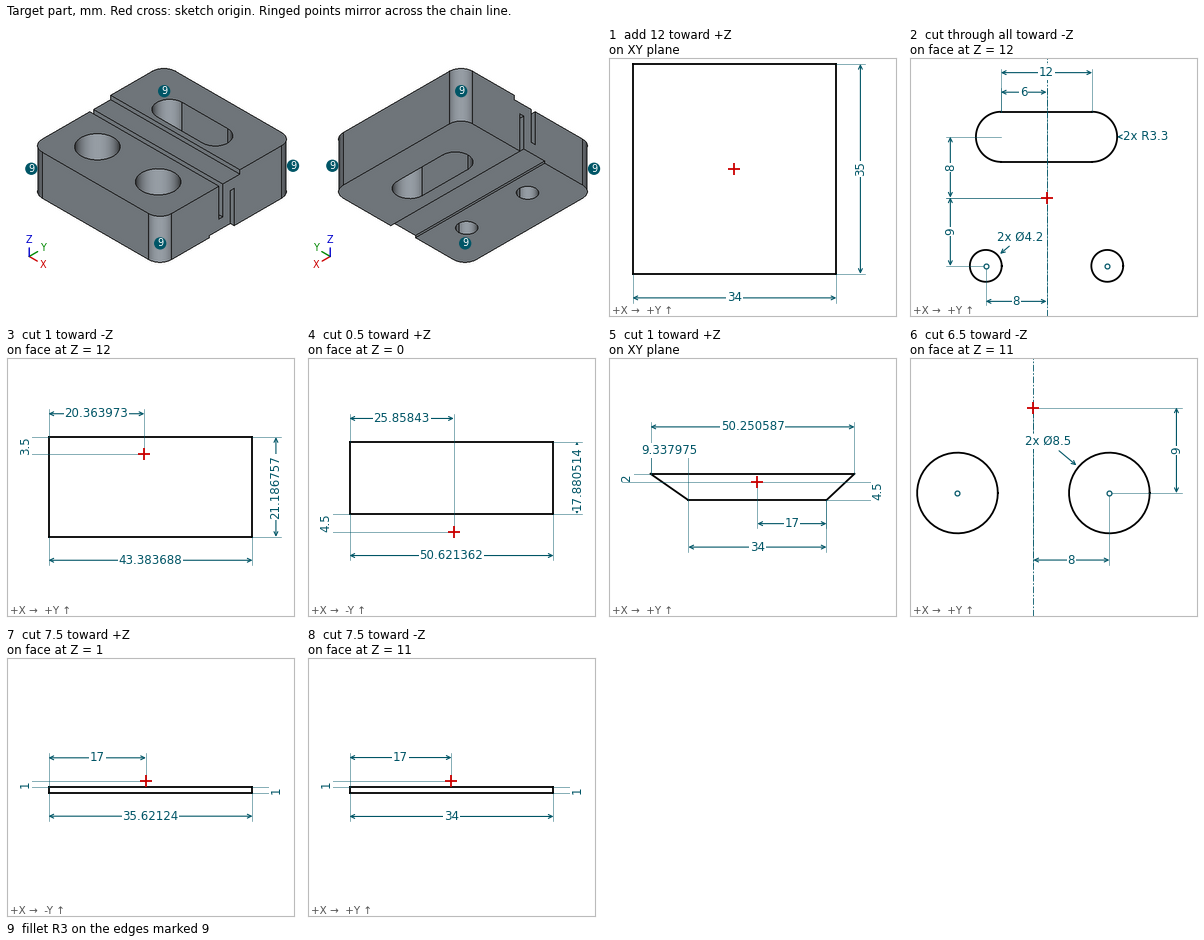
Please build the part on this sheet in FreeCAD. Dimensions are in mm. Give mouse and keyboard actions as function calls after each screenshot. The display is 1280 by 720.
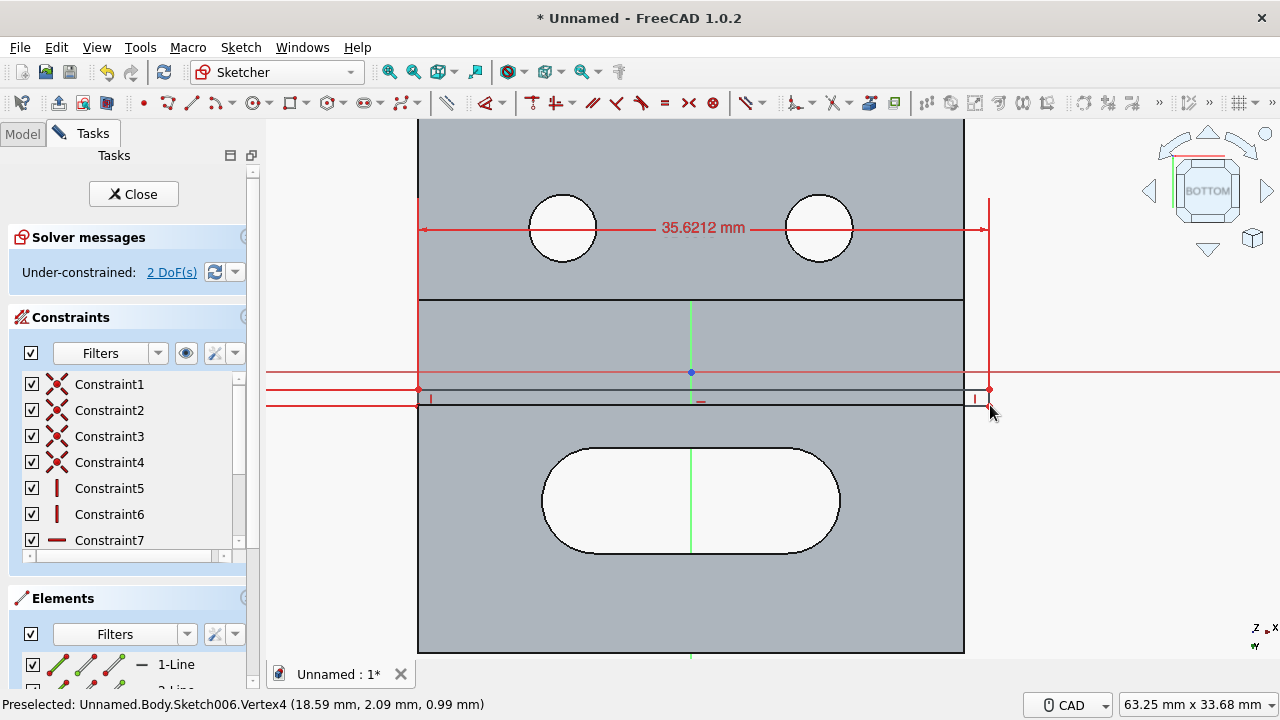
click(486, 104)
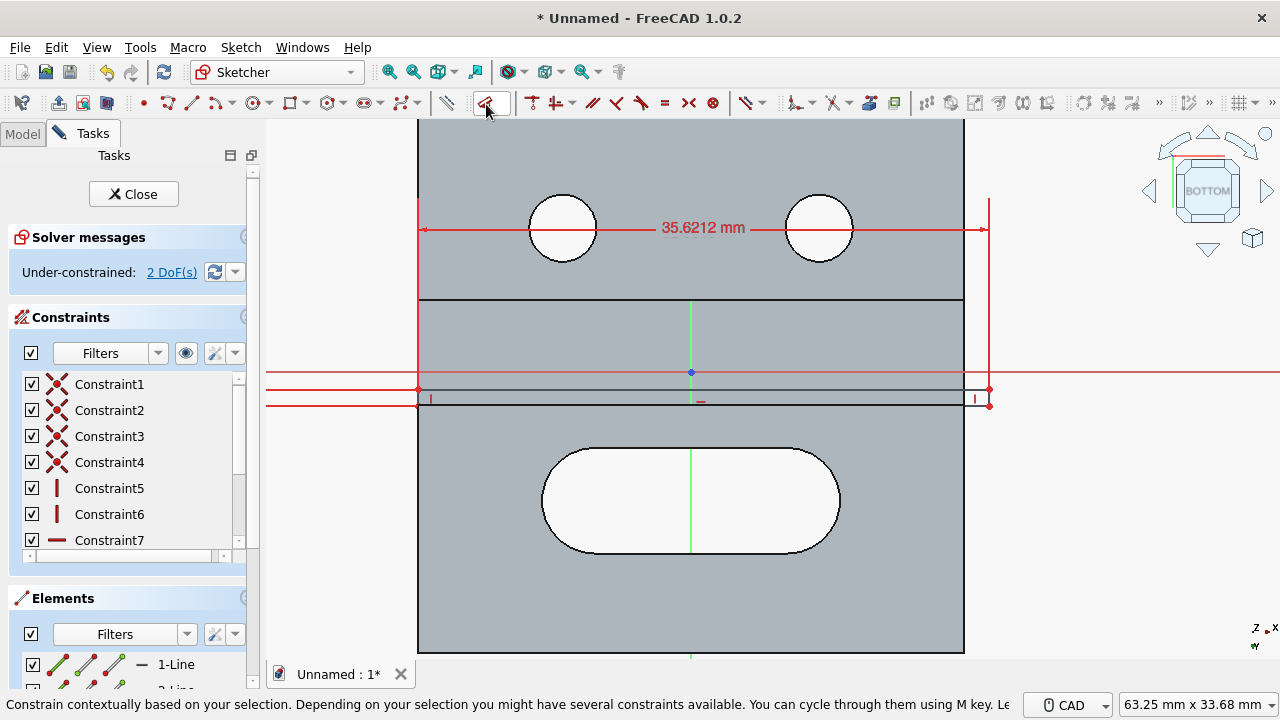
scroll(418, 390, up, 5)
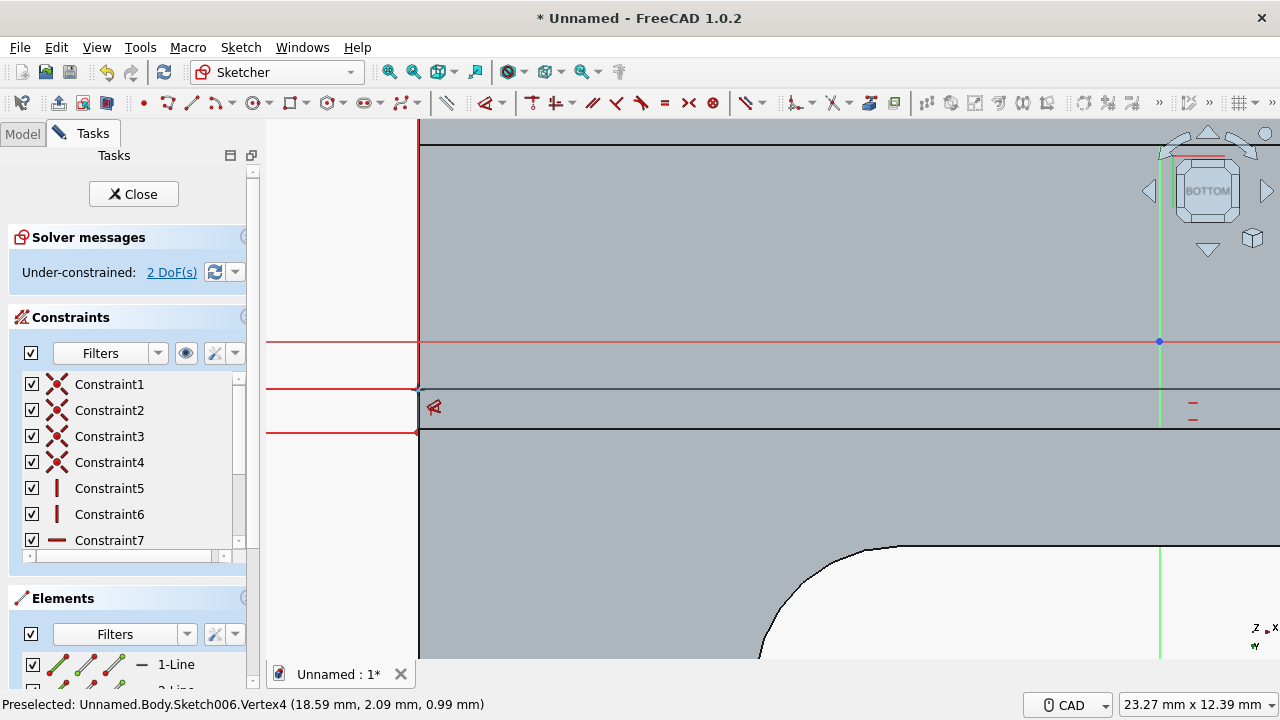
click(418, 389)
click(384, 365)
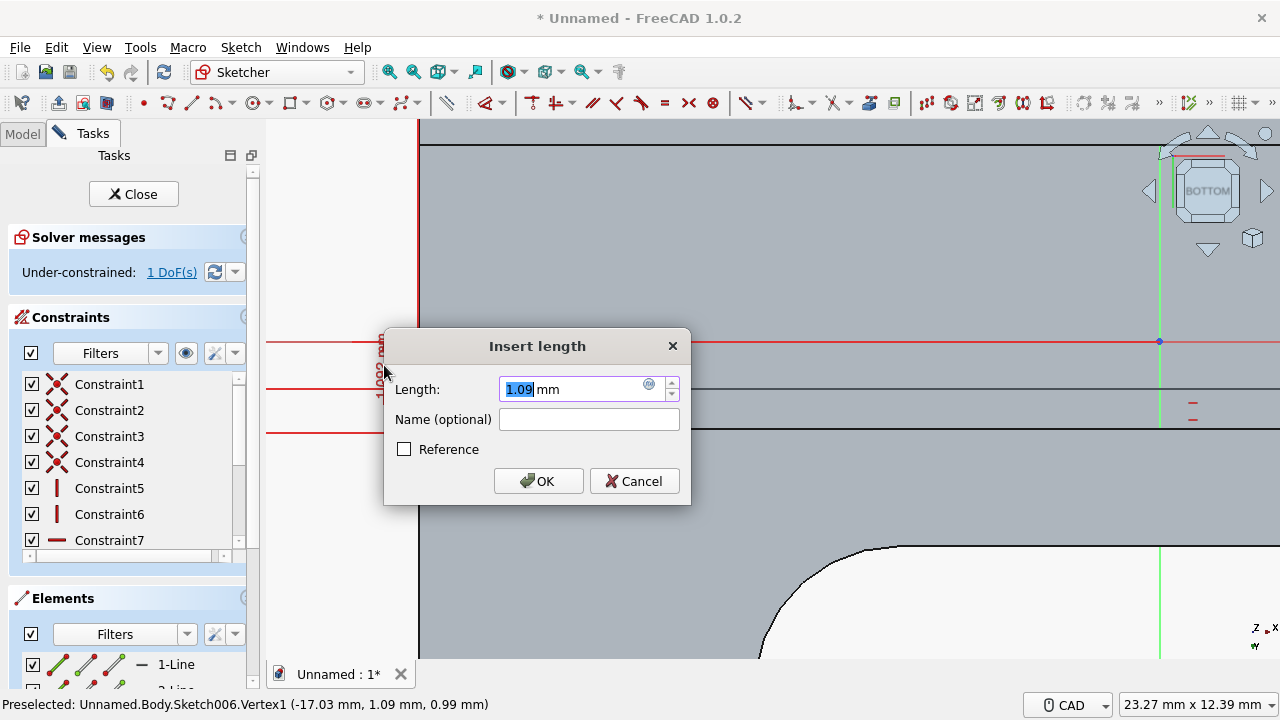
text(1)
key(Return)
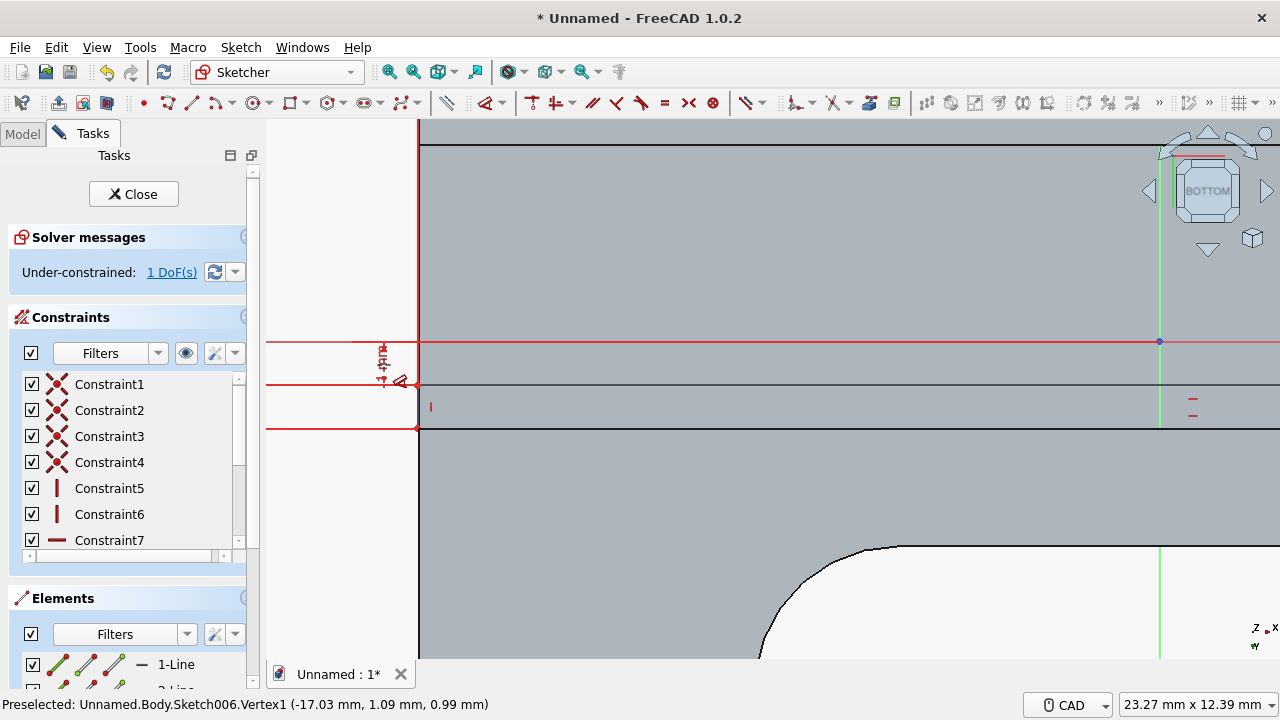
click(418, 385)
click(766, 308)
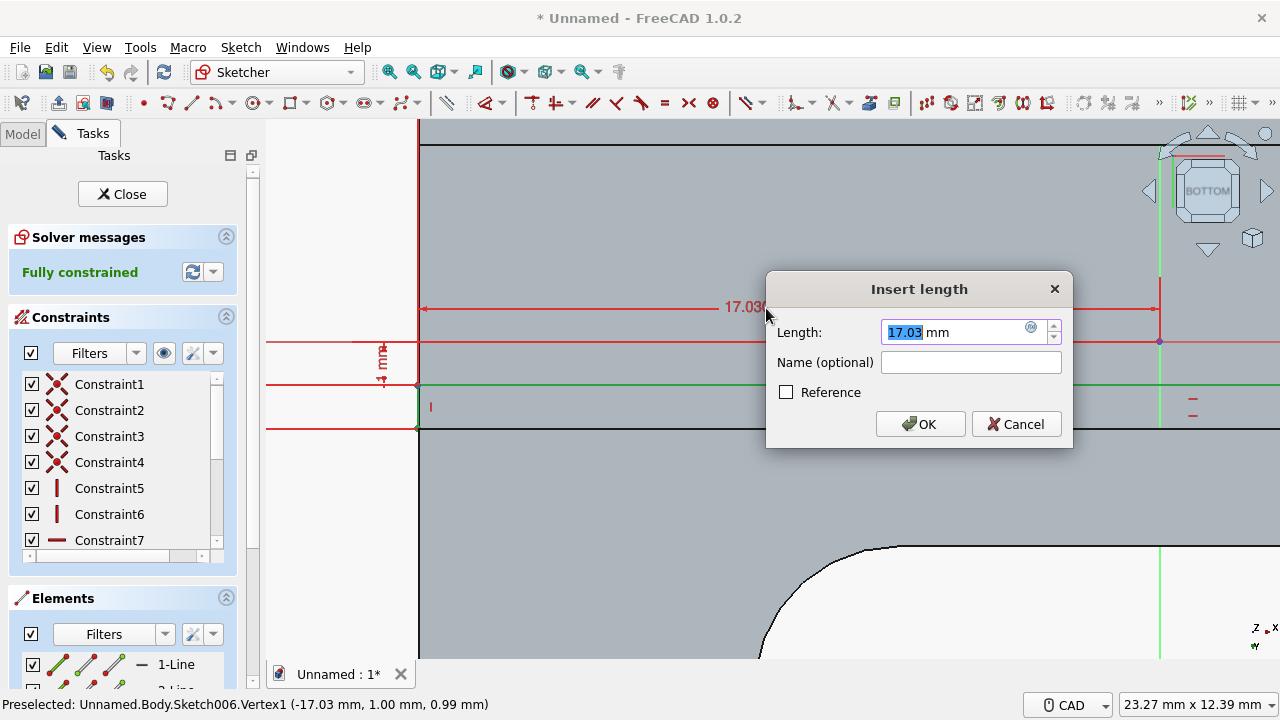
text(17)
key(Return)
key(Escape)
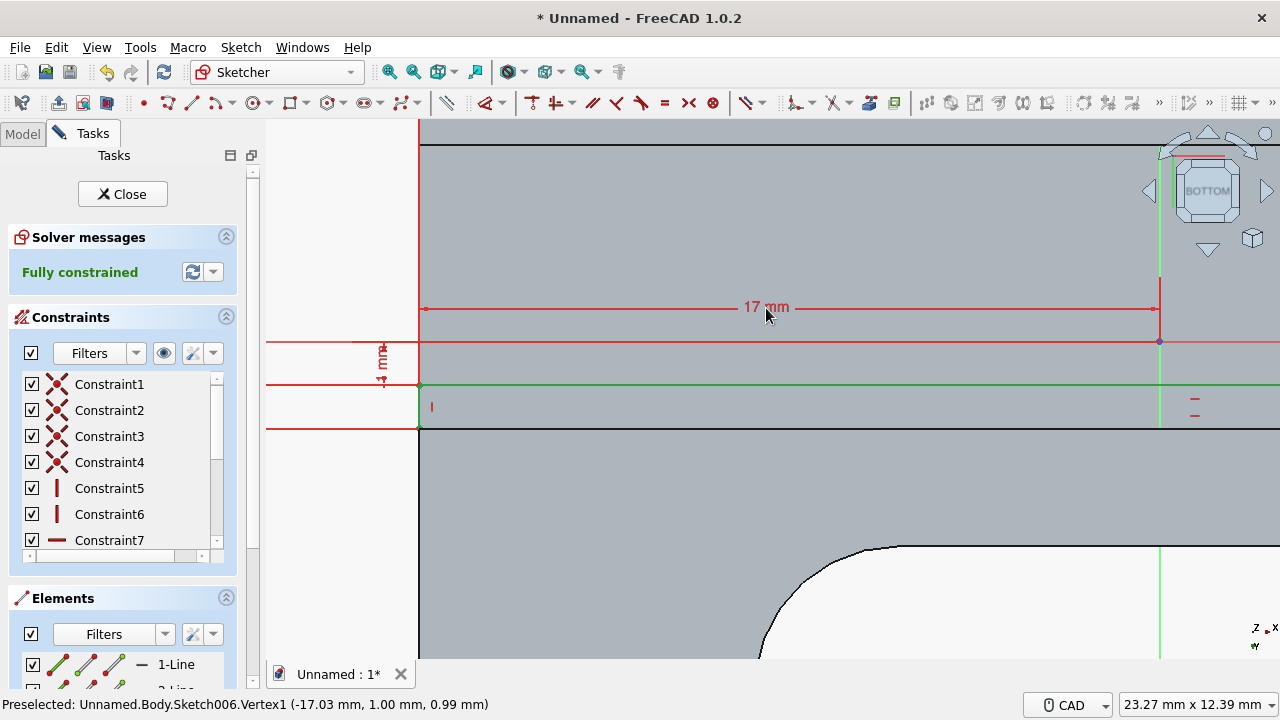
click(123, 194)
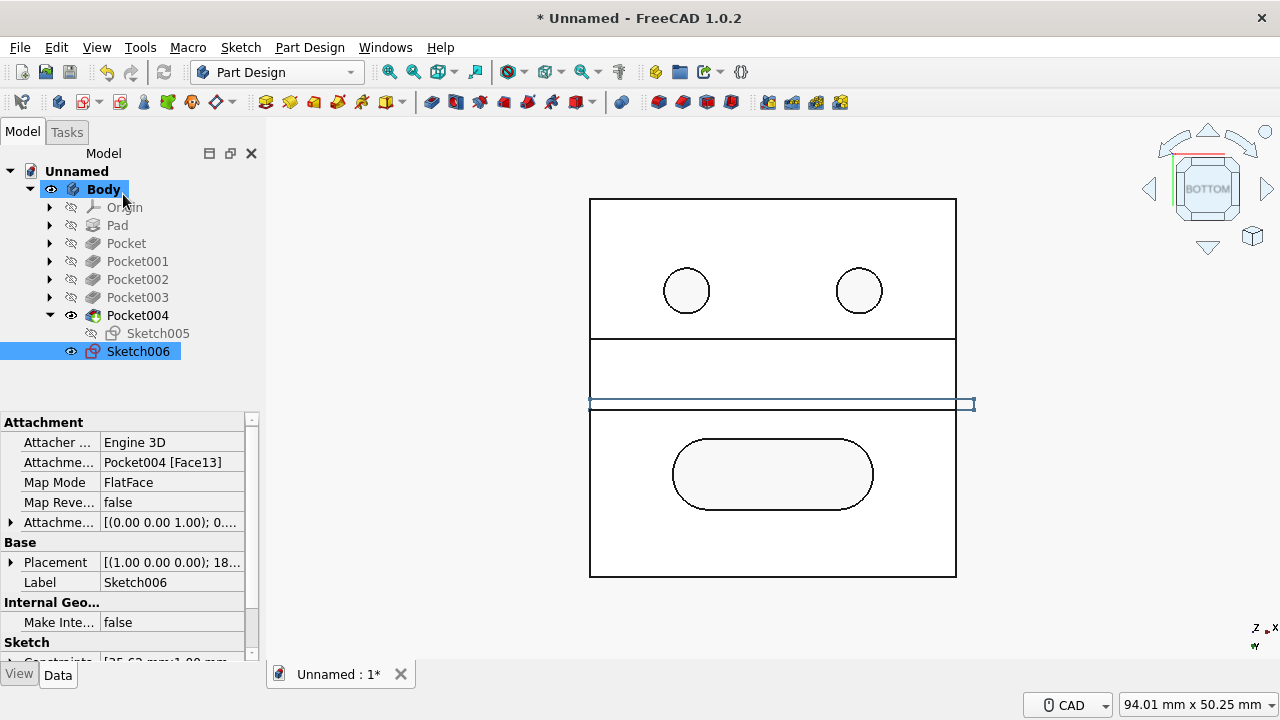
click(432, 102)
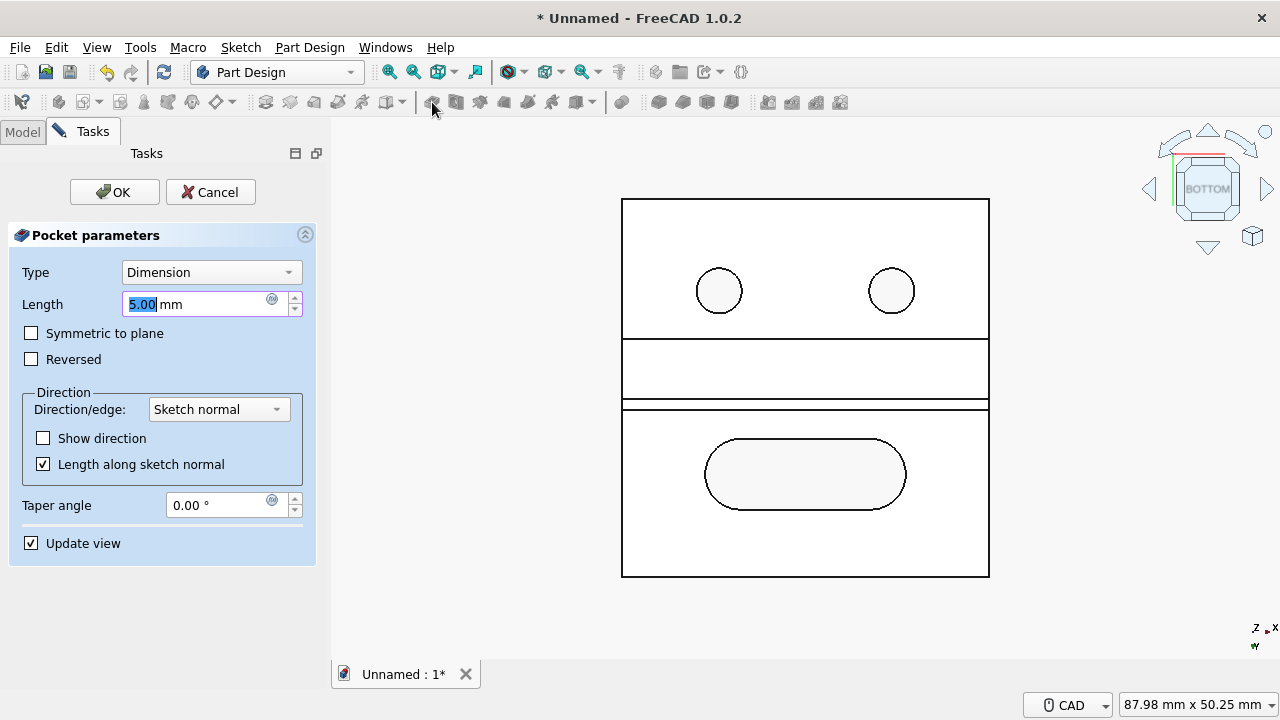
text(7.5)
key(Tab)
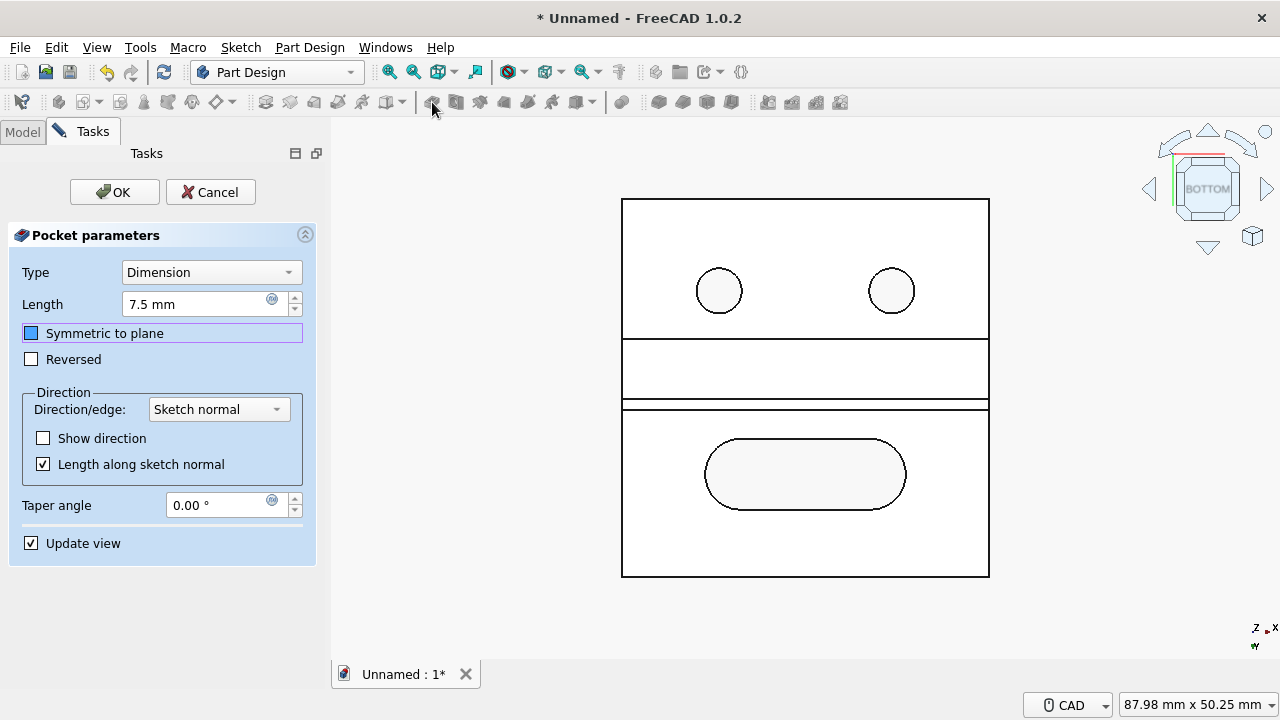
click(115, 192)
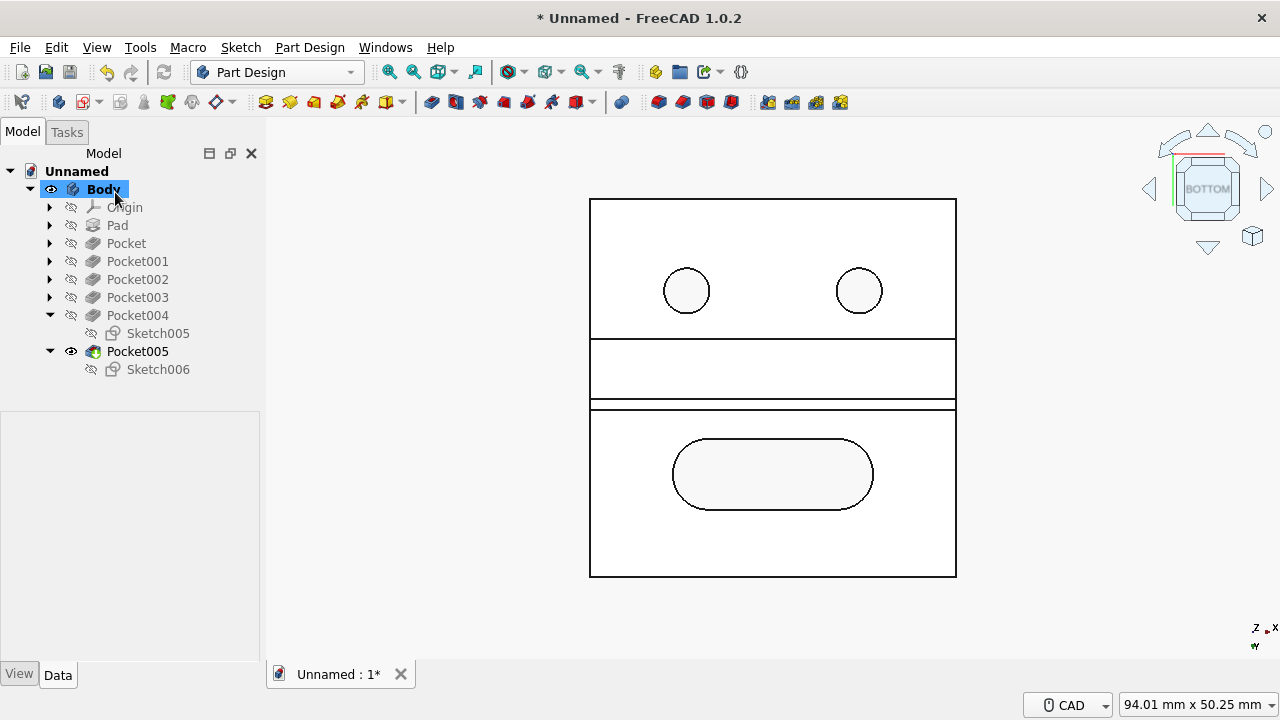
key(0)